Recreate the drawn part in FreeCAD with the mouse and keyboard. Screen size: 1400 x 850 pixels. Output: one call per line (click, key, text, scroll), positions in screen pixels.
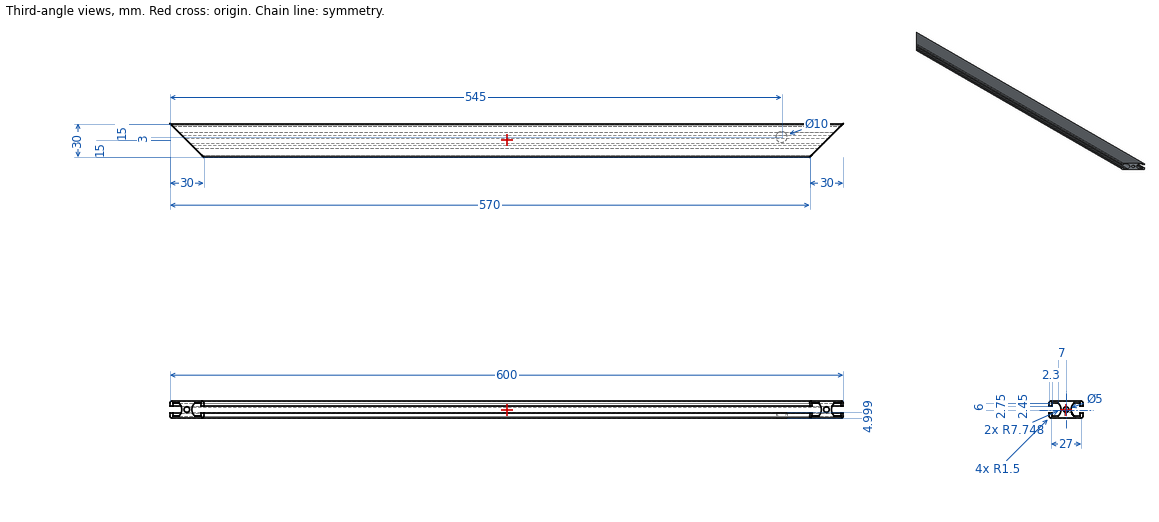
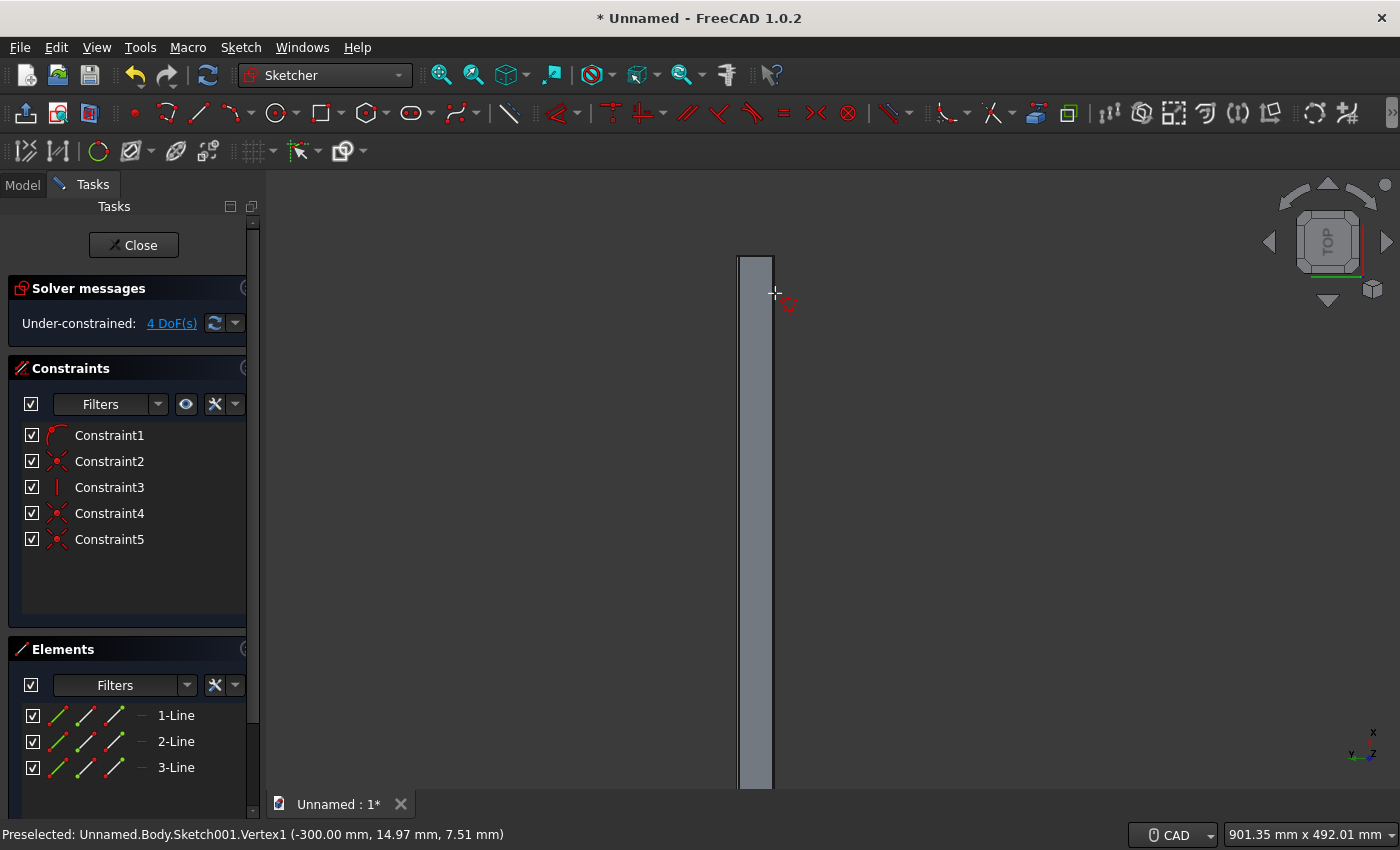
click(774, 294)
click(774, 256)
click(737, 256)
click(774, 295)
key(Escape)
key(Escape)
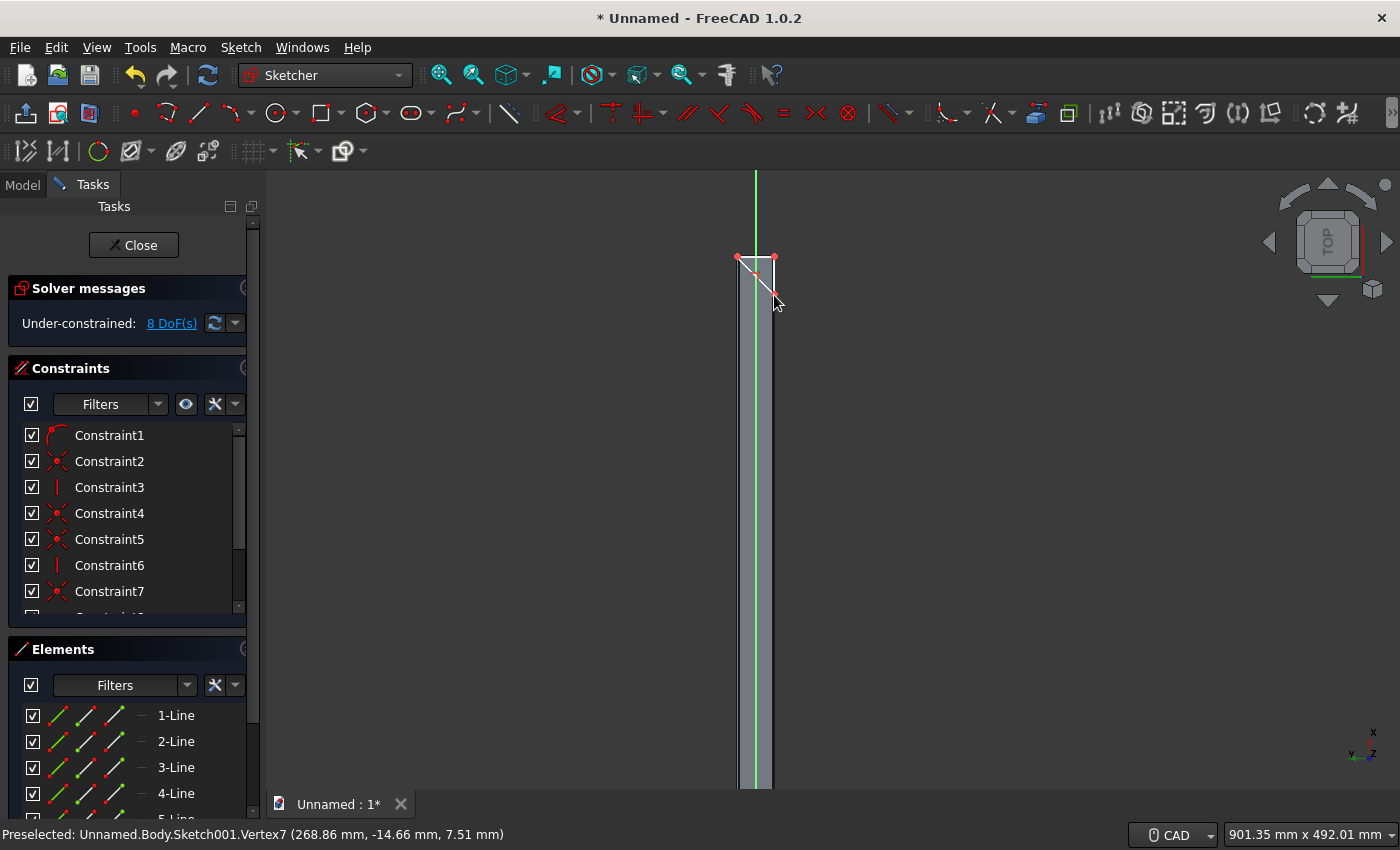
scroll(775, 292, down, 3)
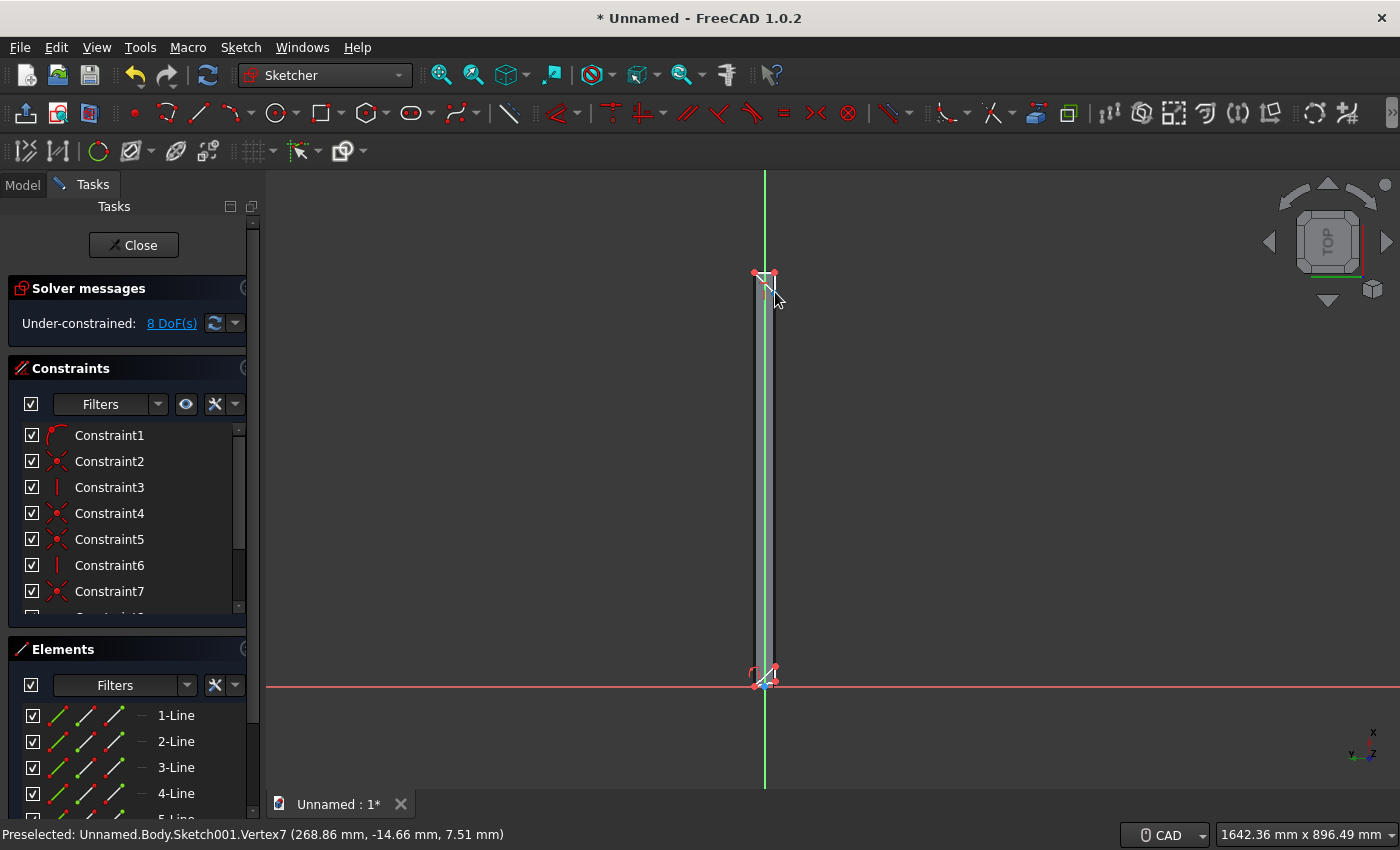
scroll(763, 685, up, 6)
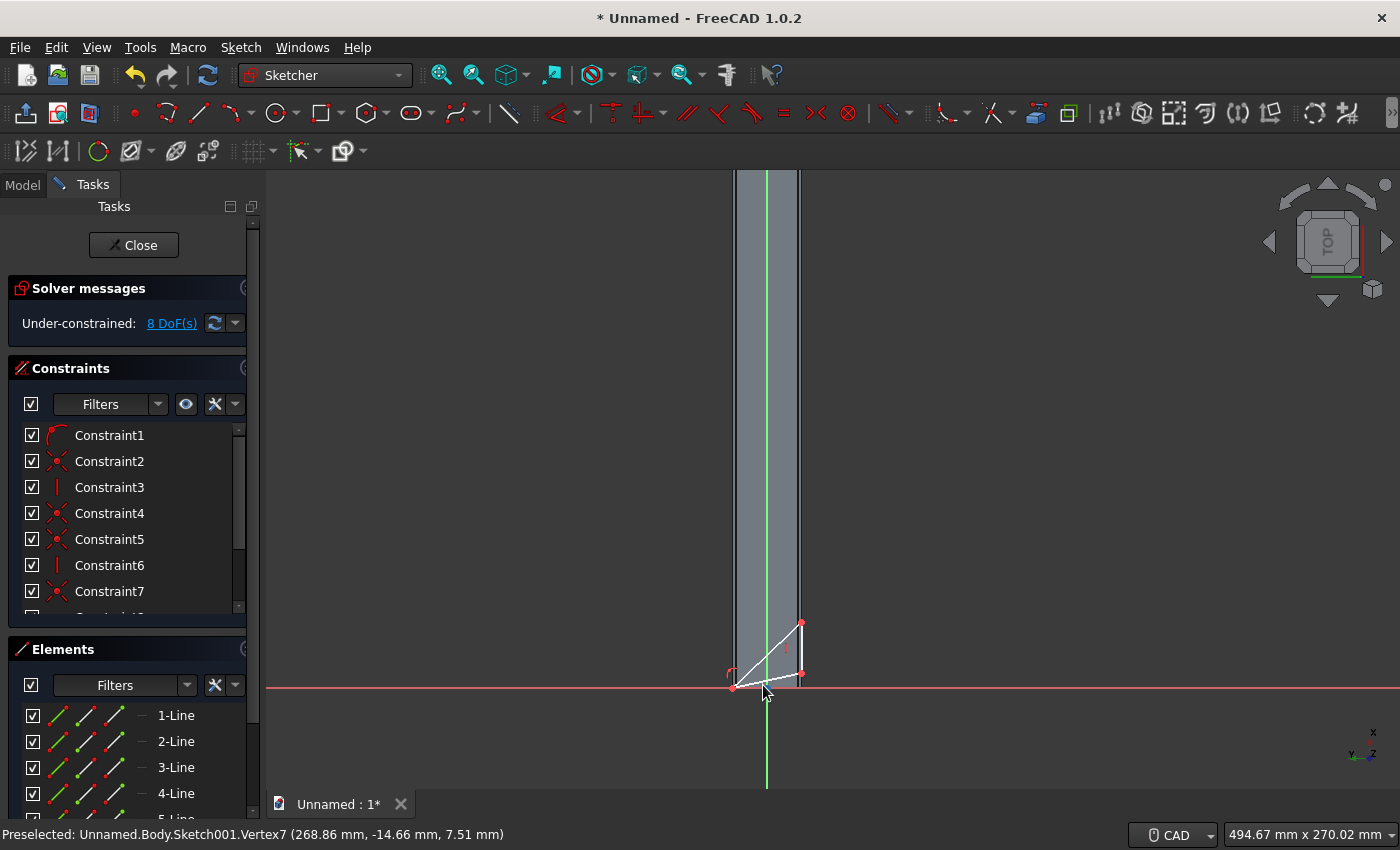
click(760, 682)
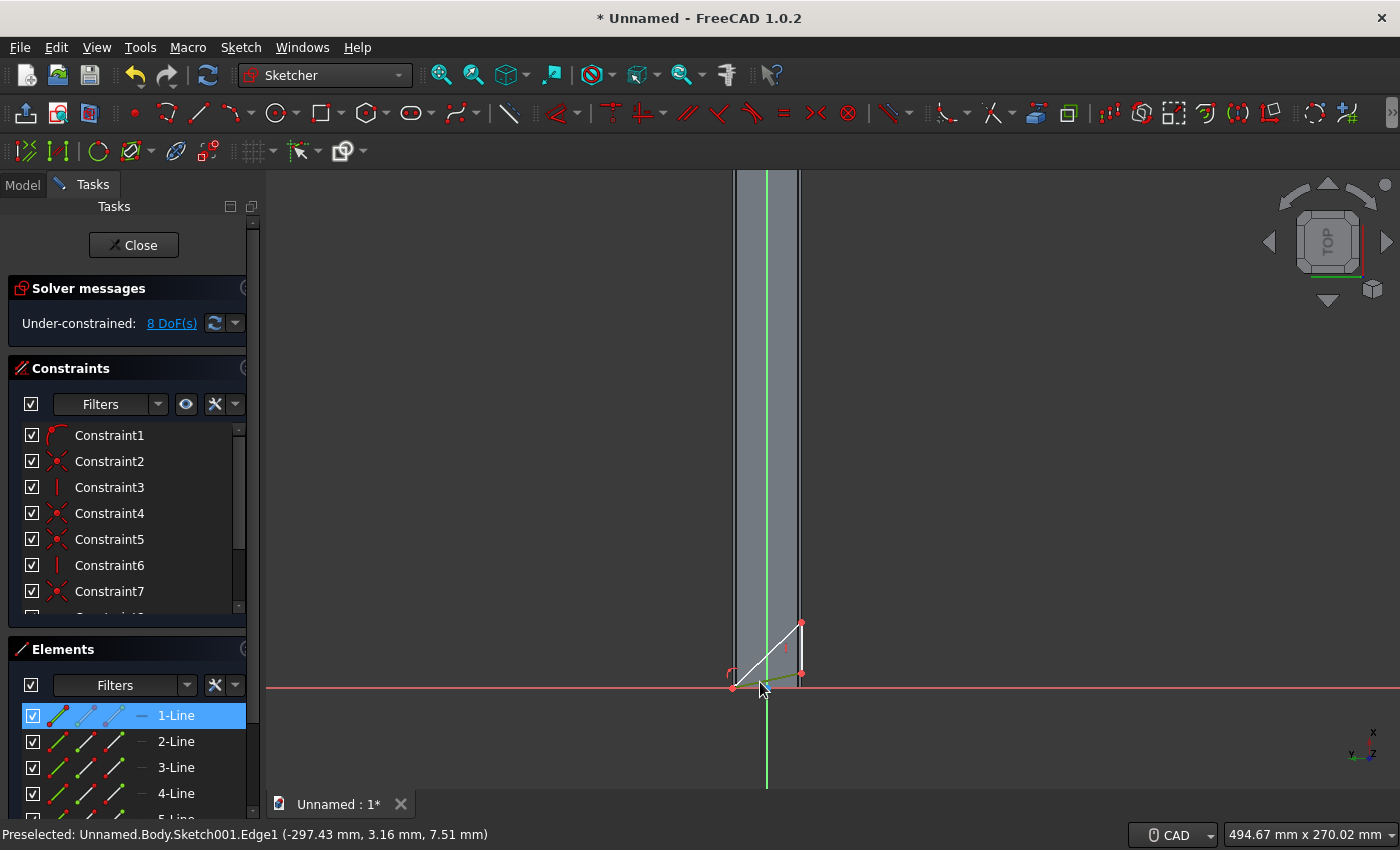
key(h)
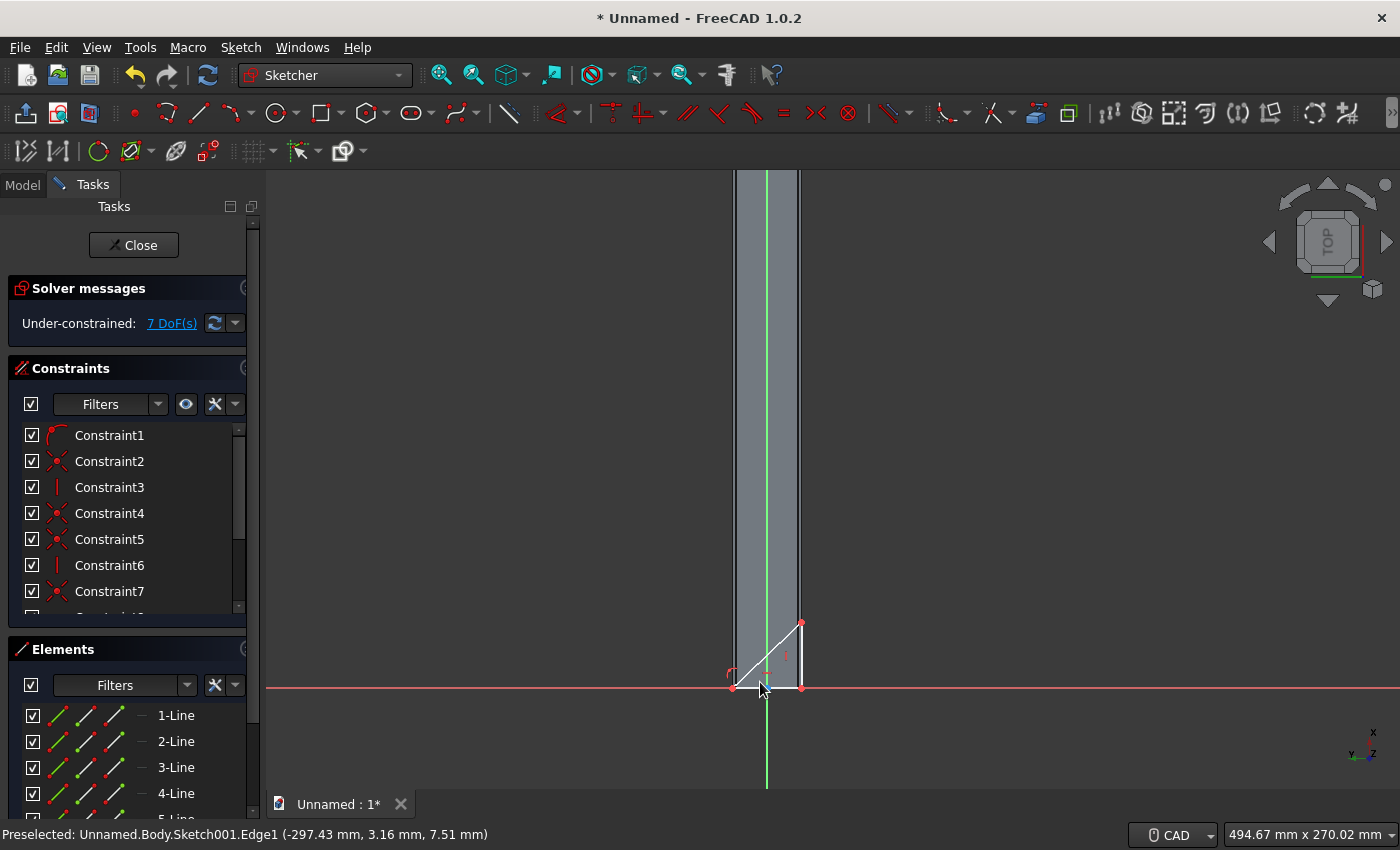
key(d)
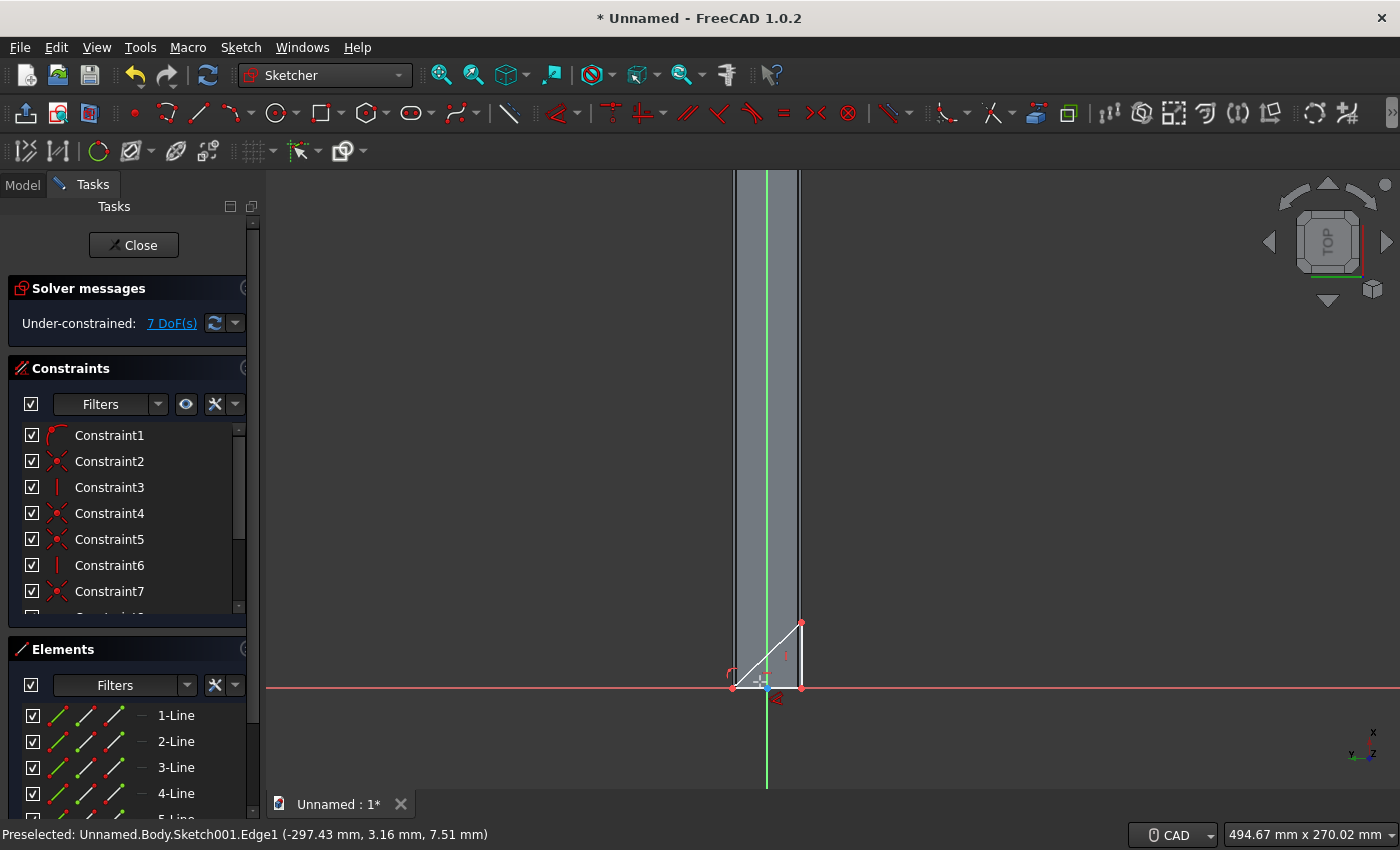
click(754, 688)
click(751, 722)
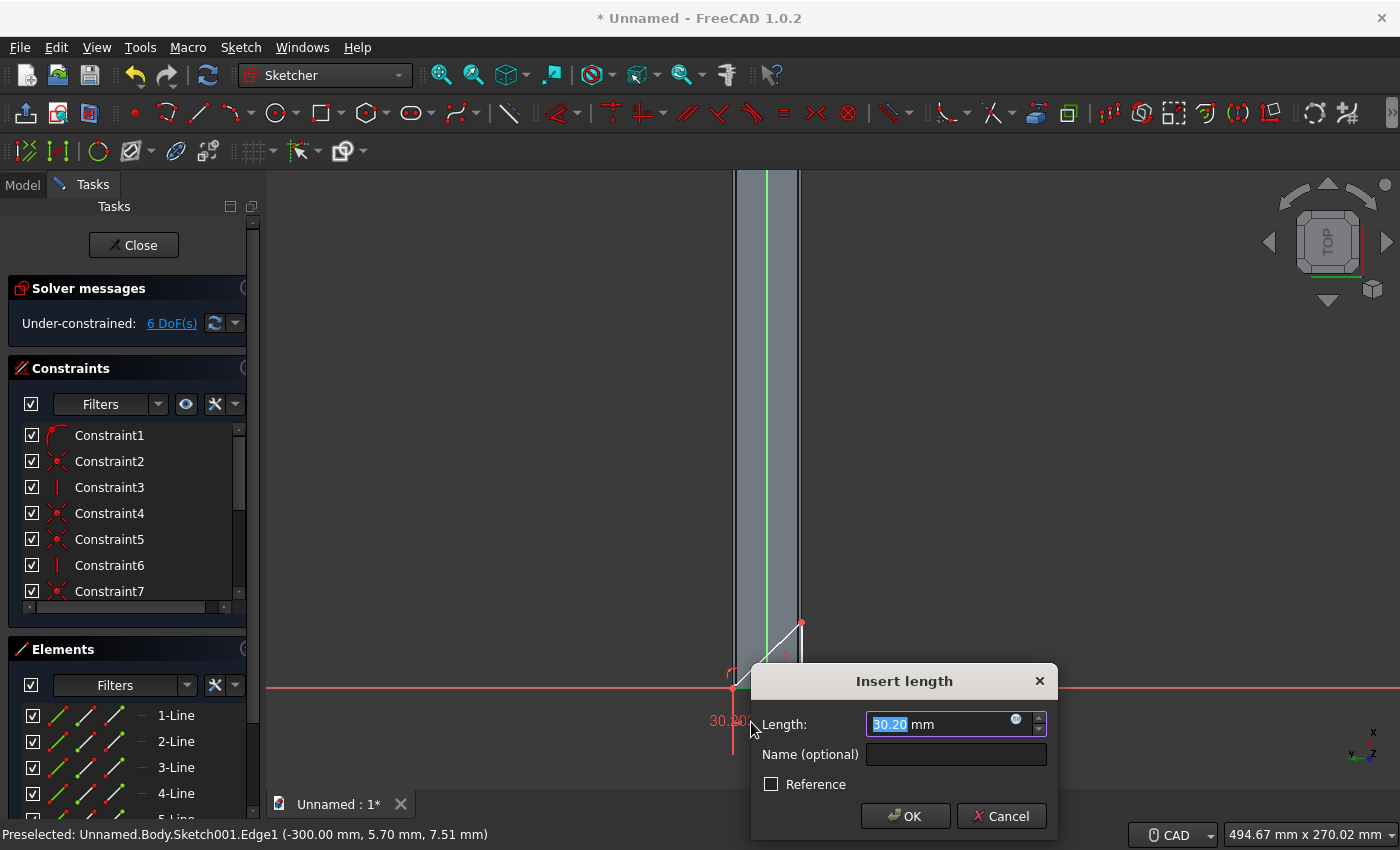
text(30)
key(Return)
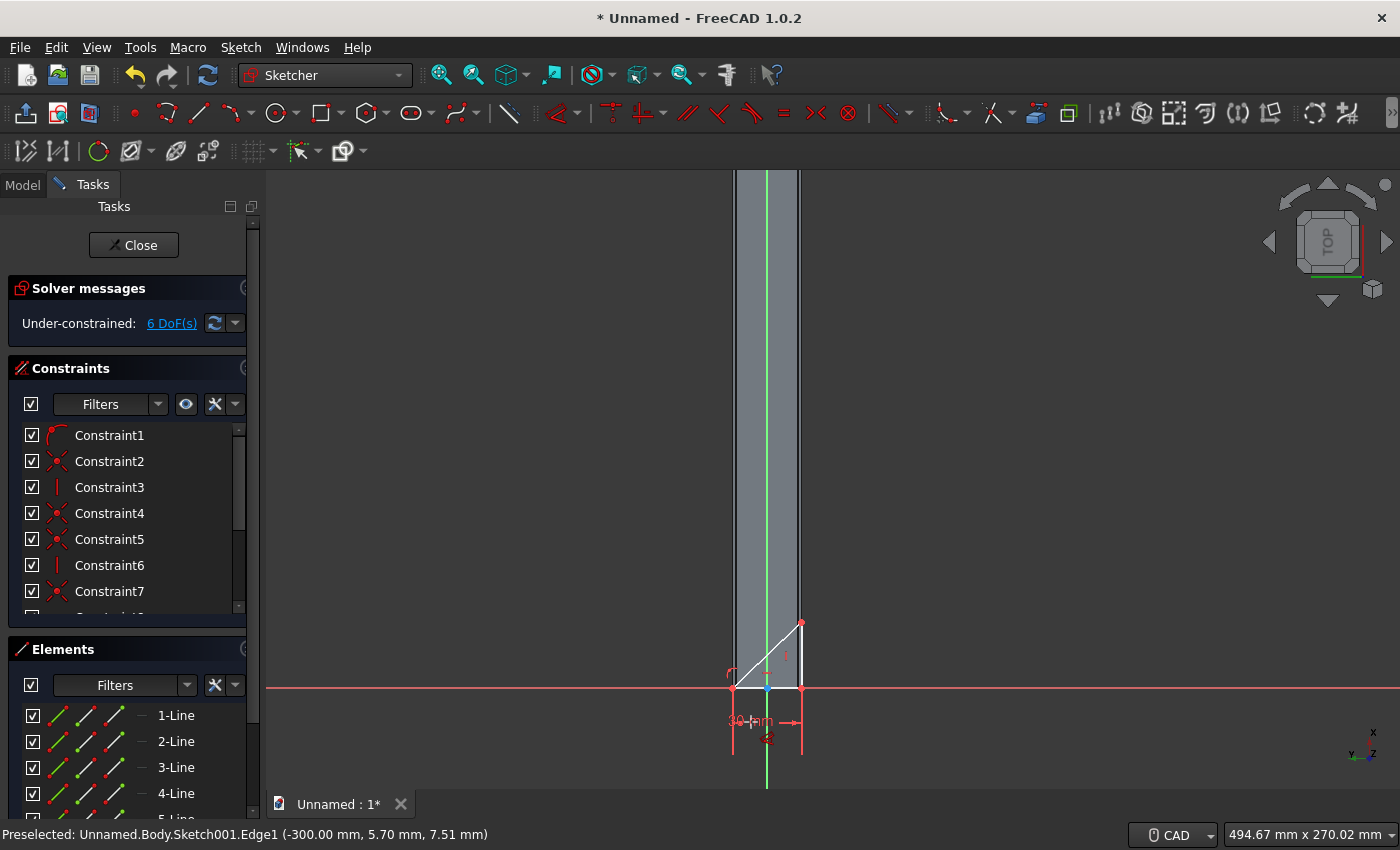
click(802, 668)
click(836, 655)